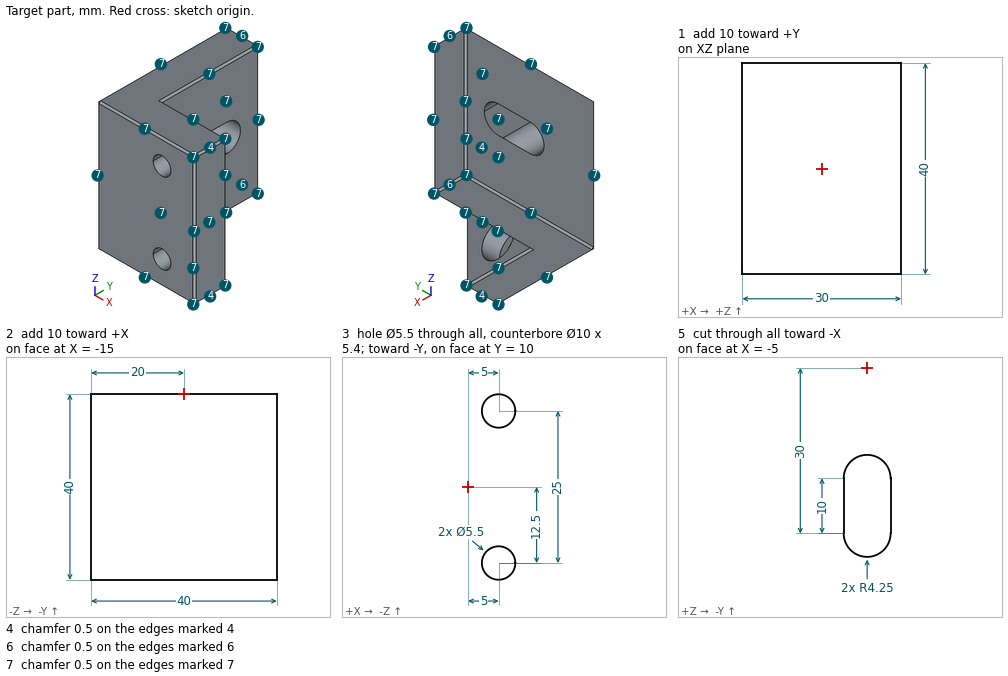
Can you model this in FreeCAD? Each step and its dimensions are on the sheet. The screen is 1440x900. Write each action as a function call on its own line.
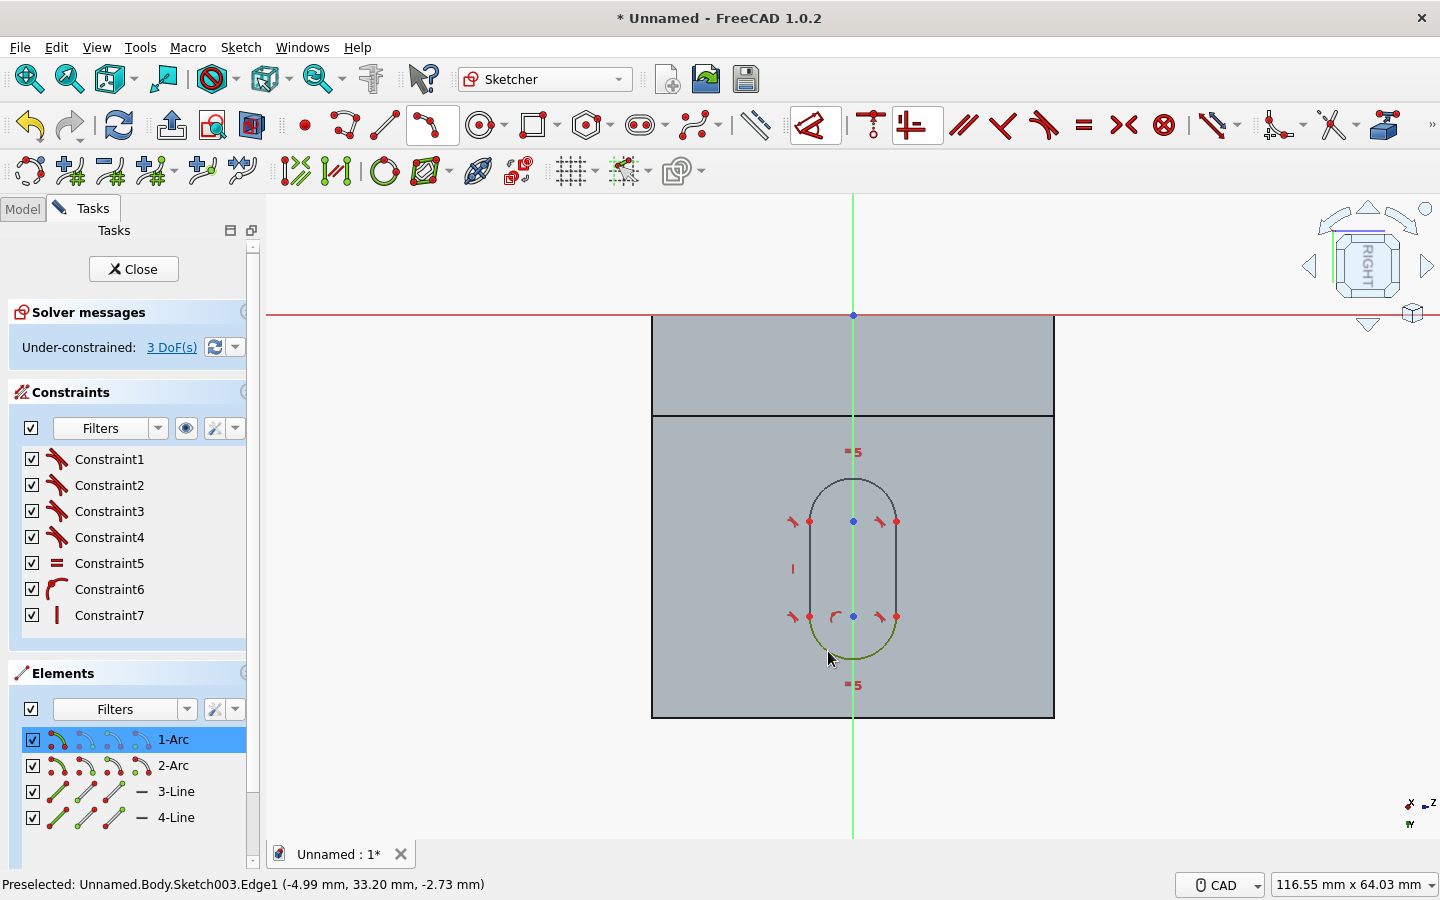
click(836, 126)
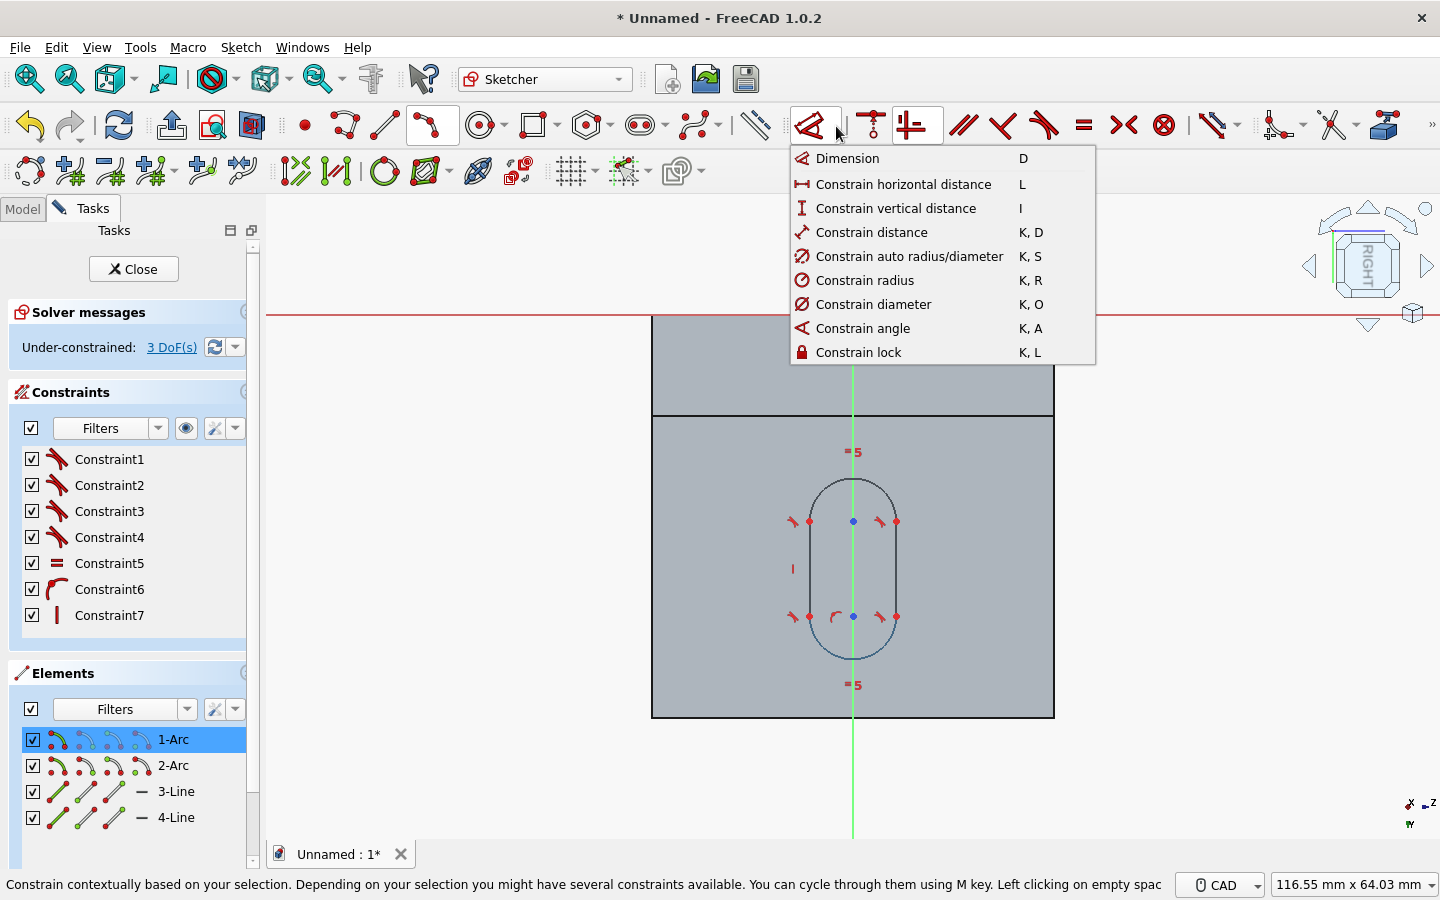
click(943, 280)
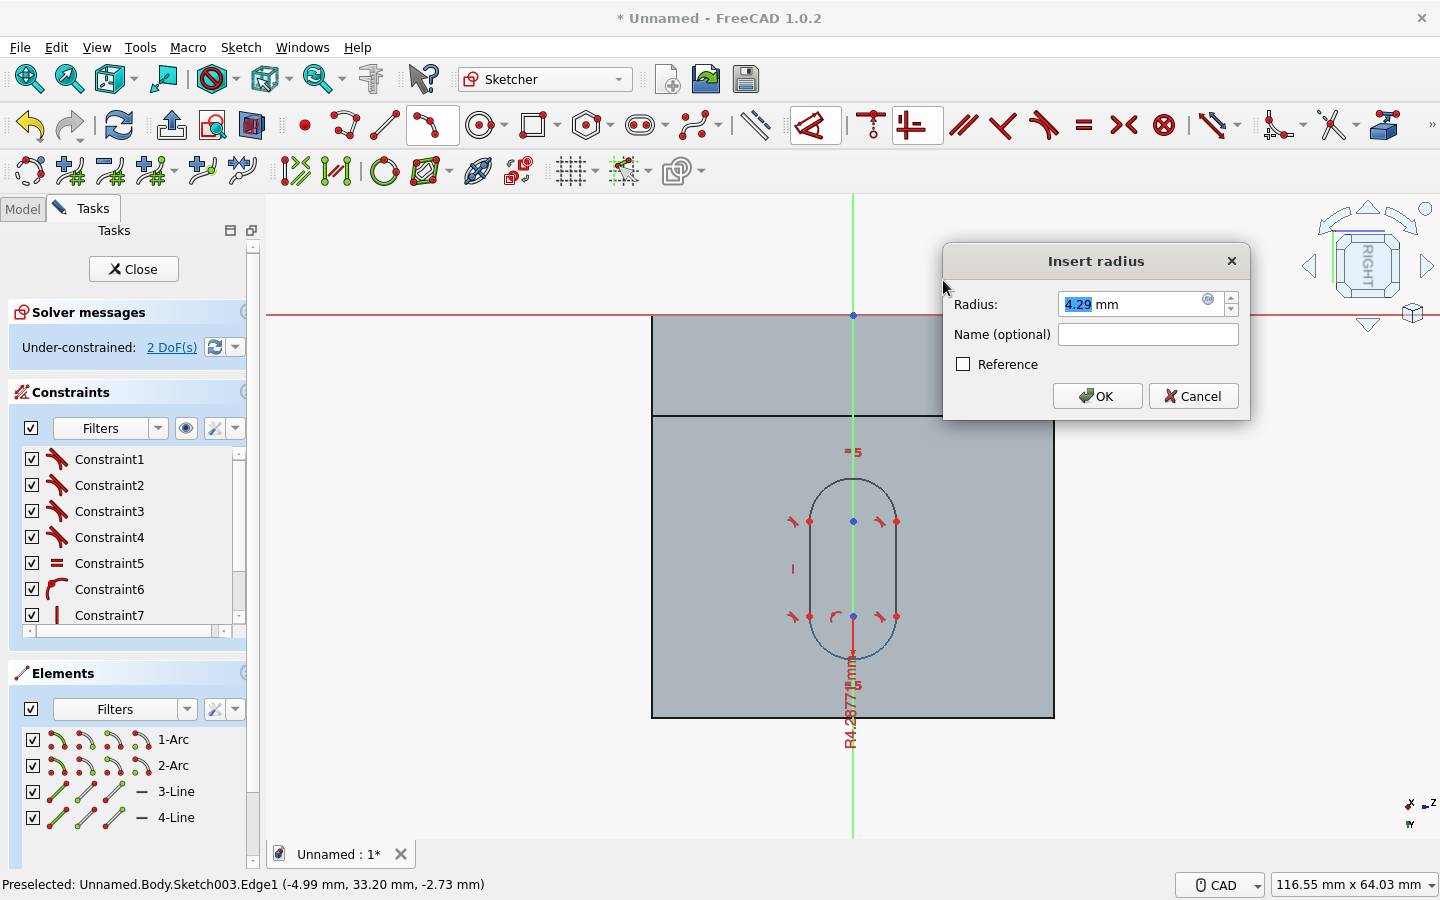
text(4.25)
key(Return)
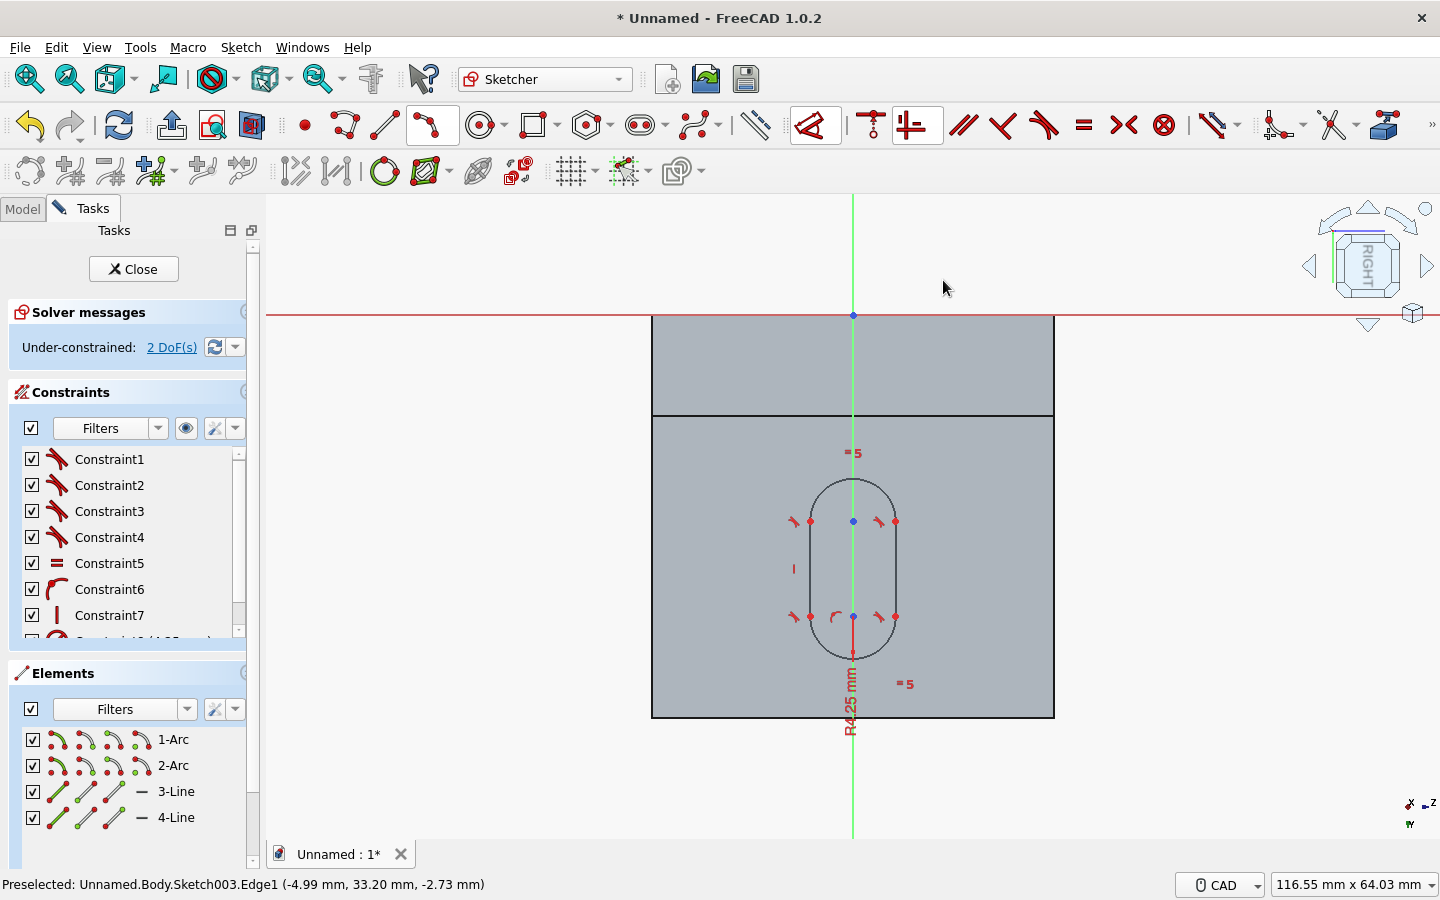
click(810, 588)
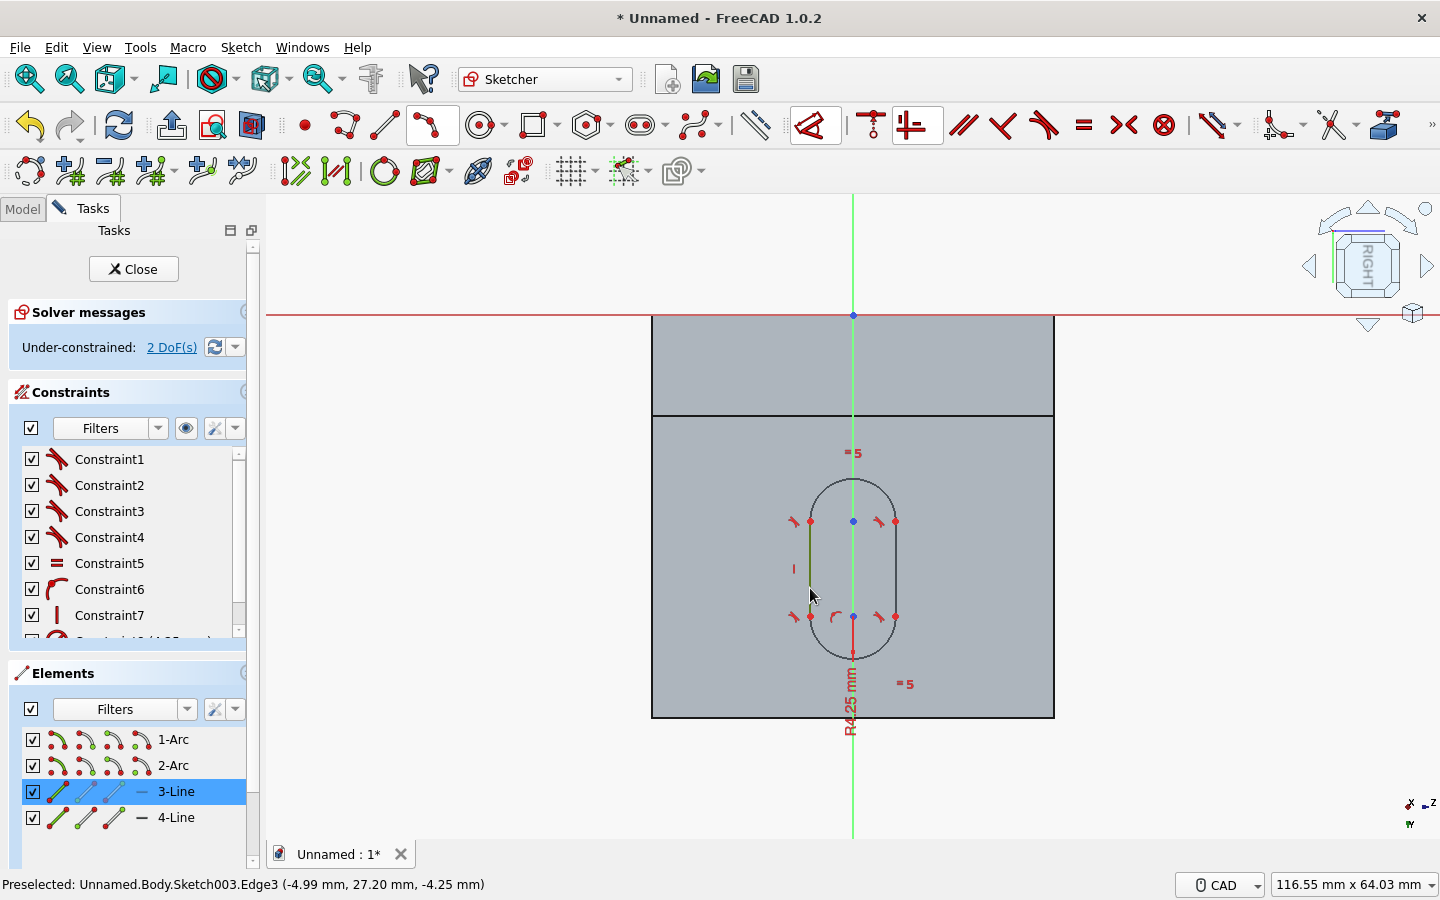
key(i)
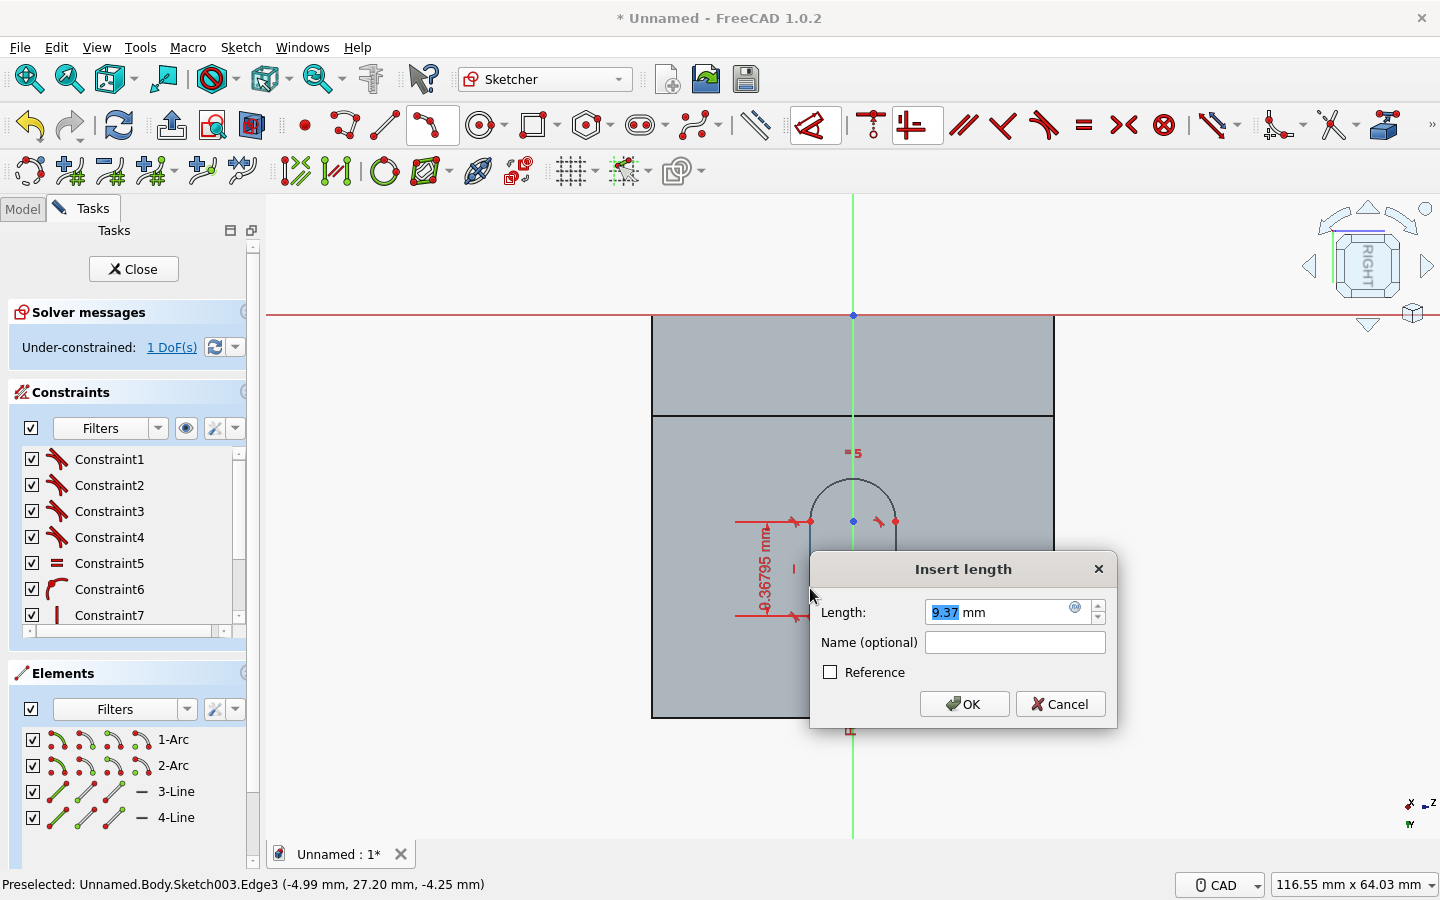
text(10)
key(Return)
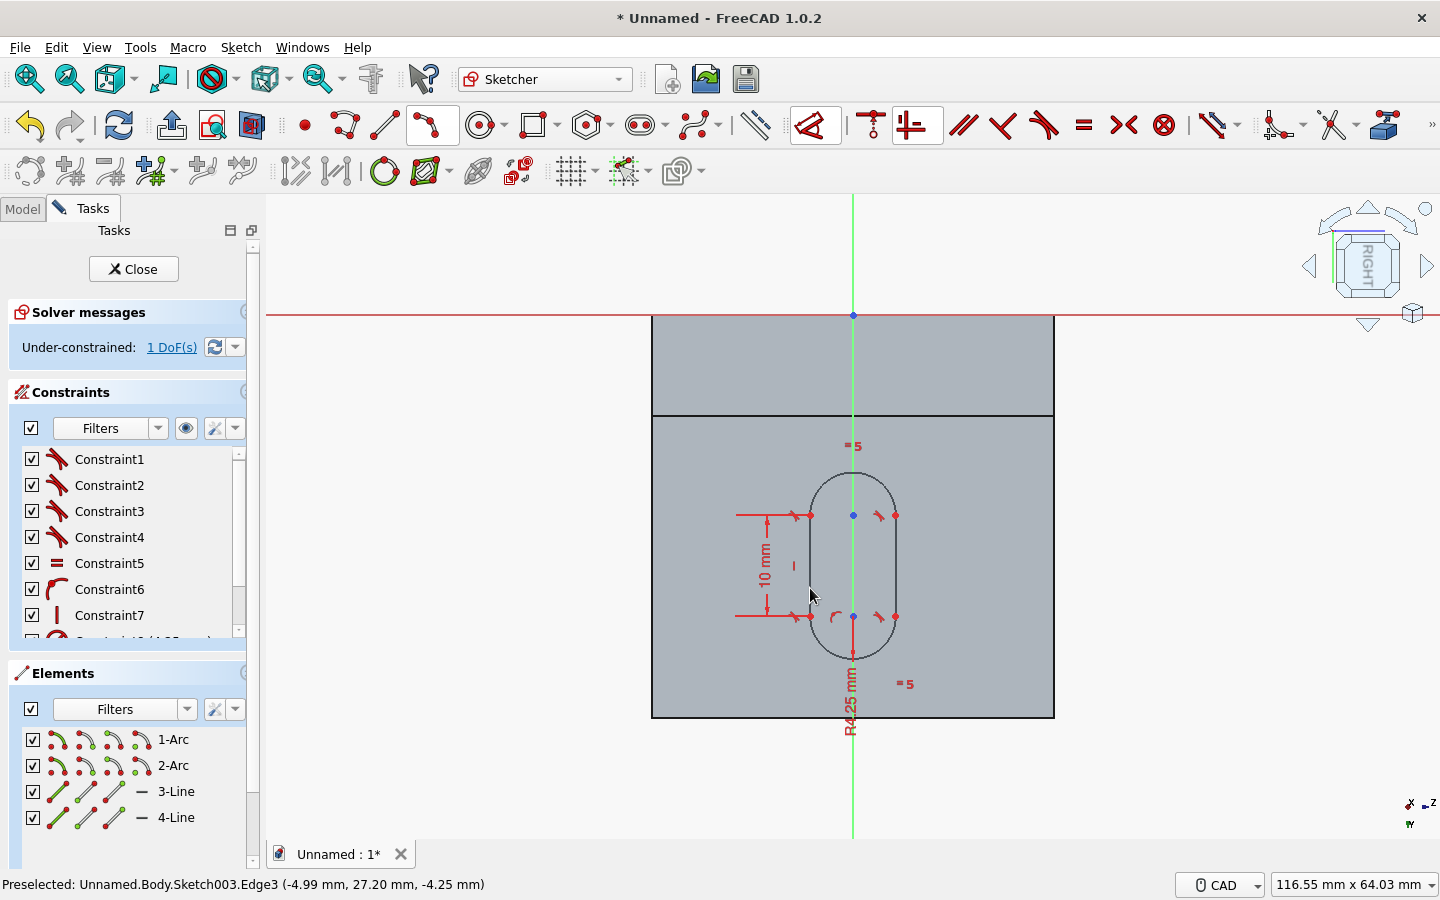
click(810, 616)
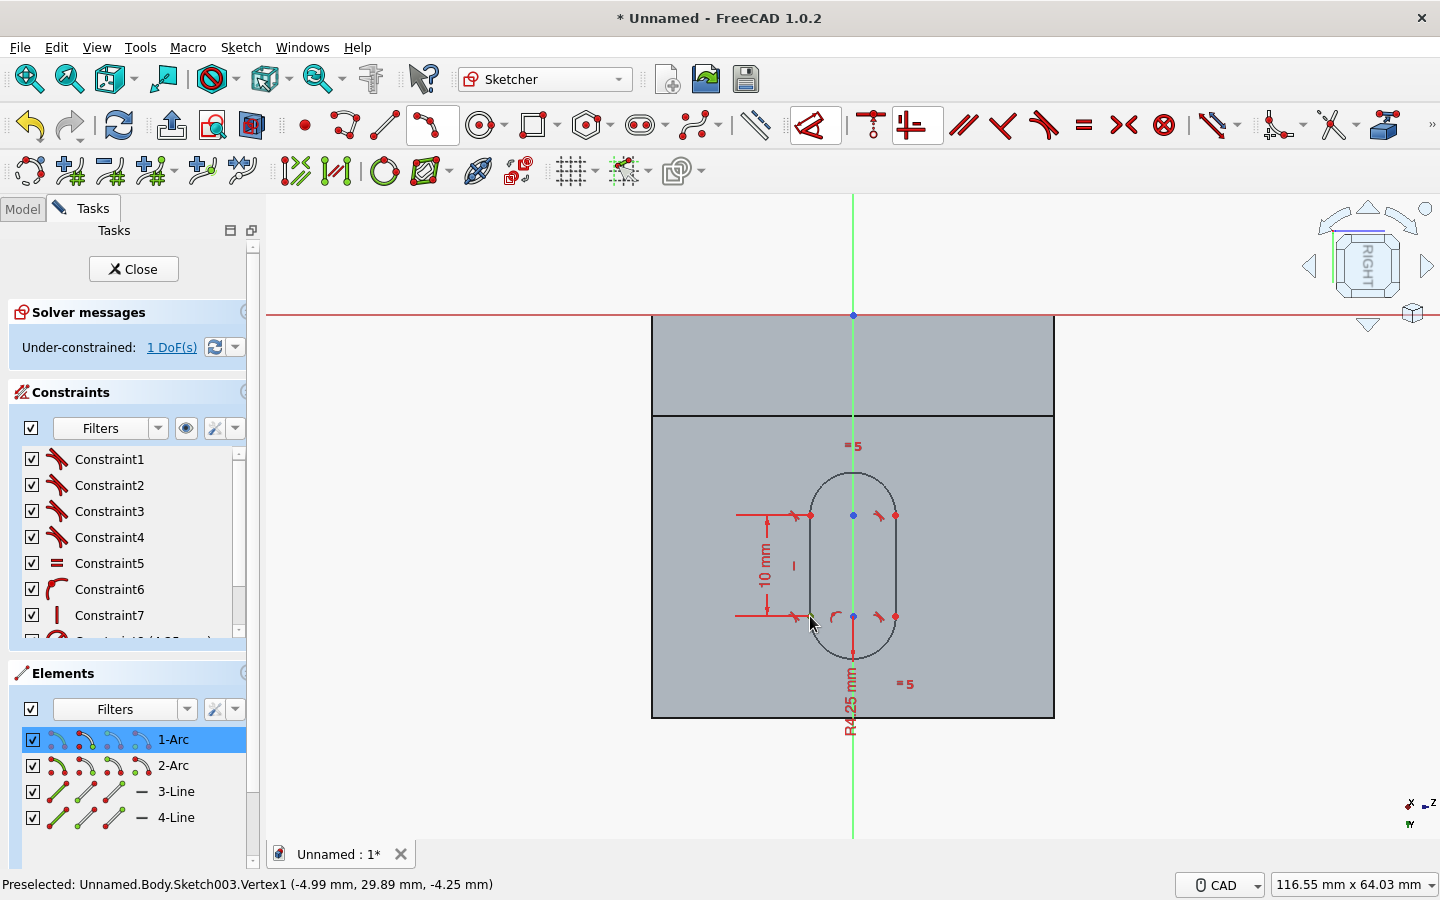
click(836, 126)